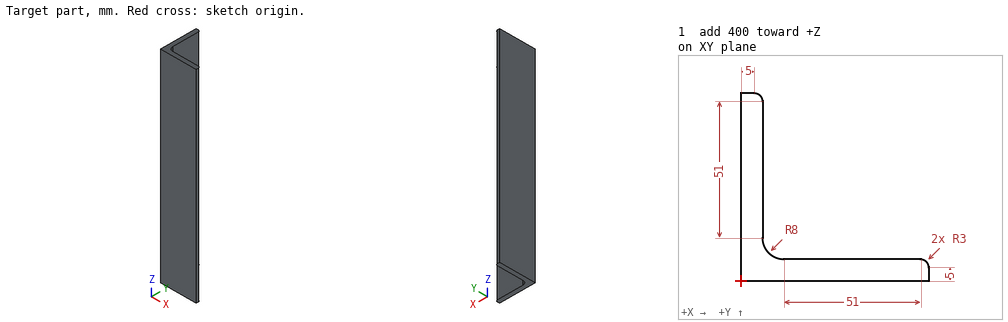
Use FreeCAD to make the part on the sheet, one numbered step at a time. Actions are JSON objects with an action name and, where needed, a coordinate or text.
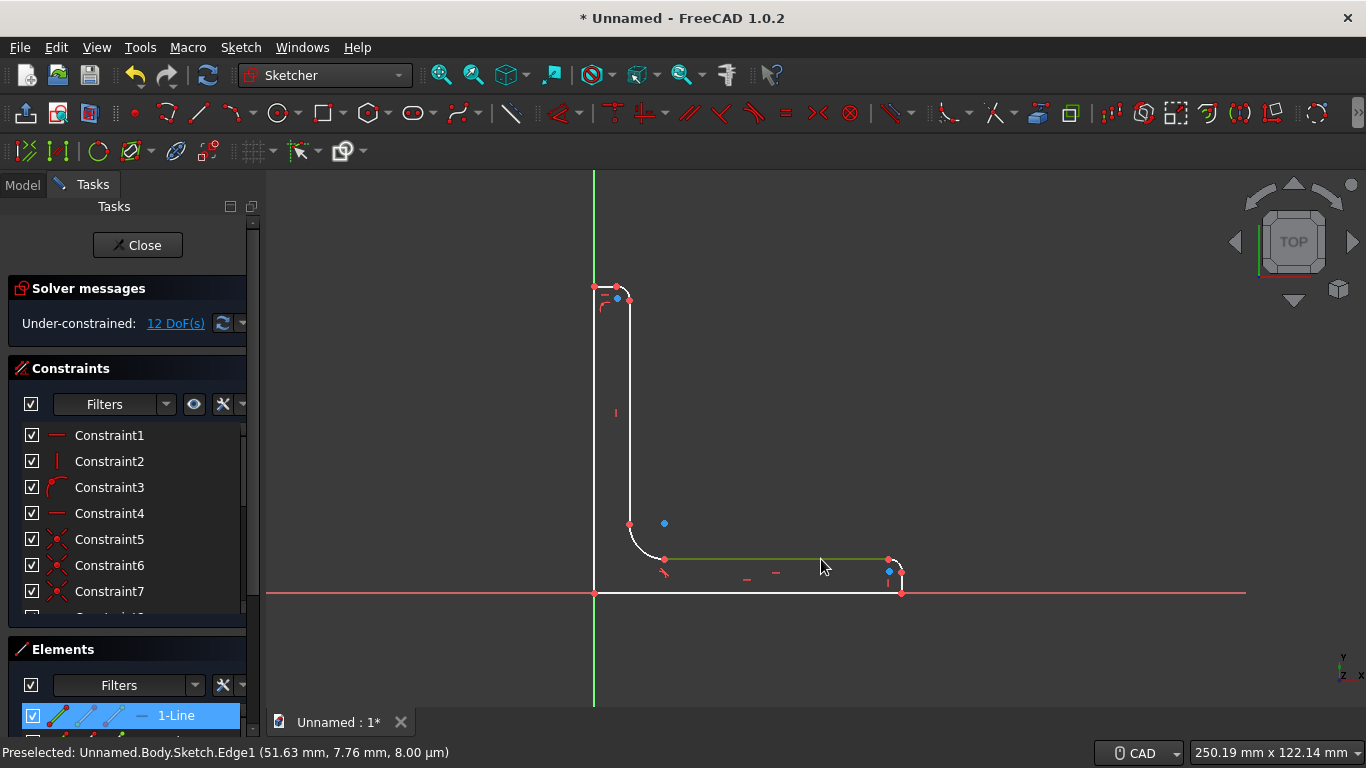
{"action": "scroll", "coordinate": [898, 563], "scroll_direction": "up", "scroll_amount": 2}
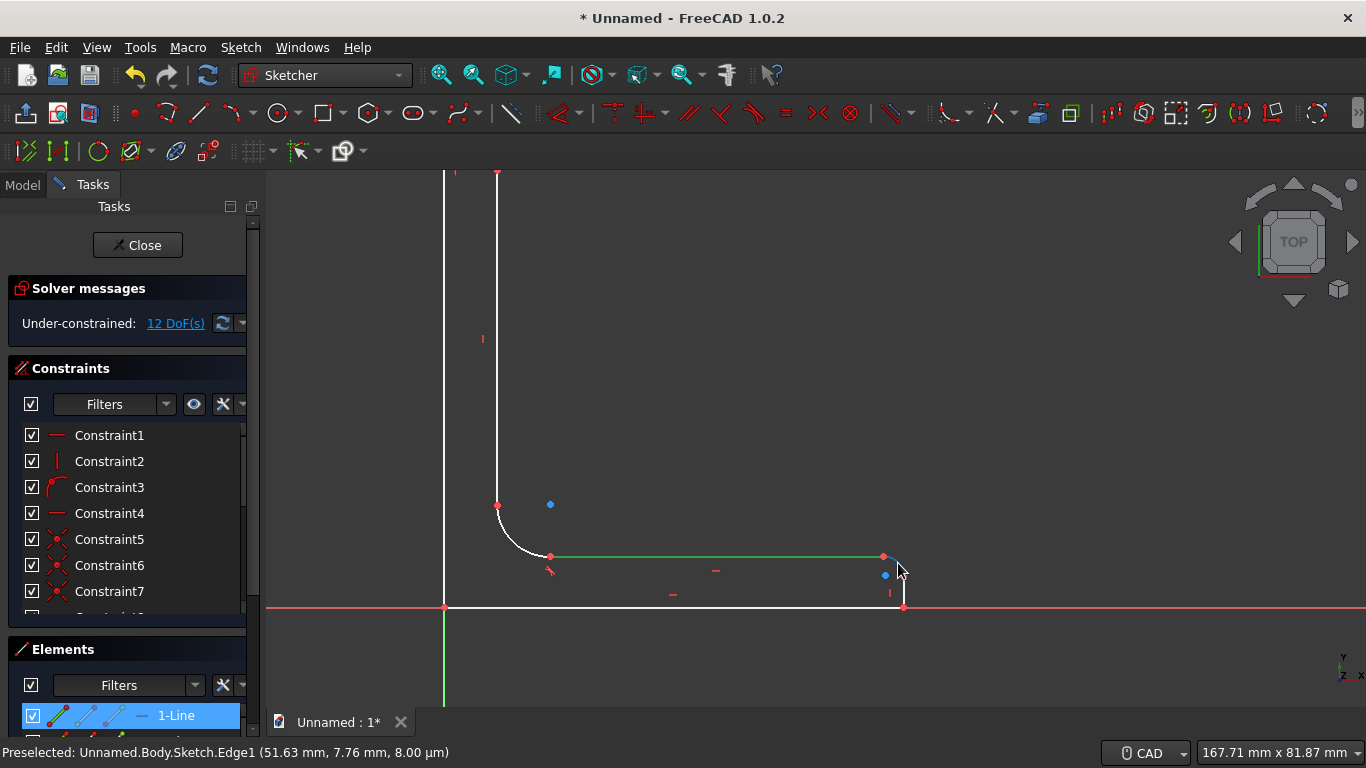
{"action": "left_click", "coordinate": [898, 562]}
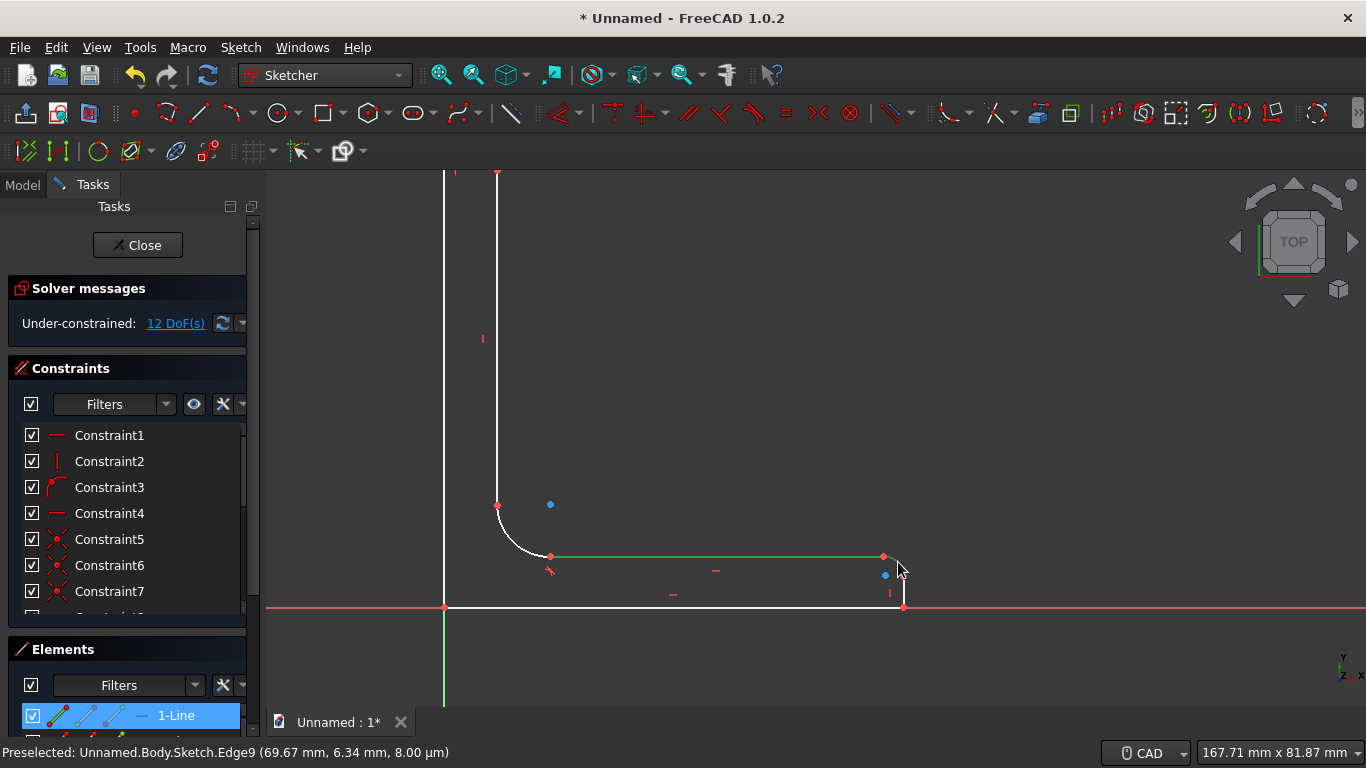
{"action": "left_click", "coordinate": [754, 114]}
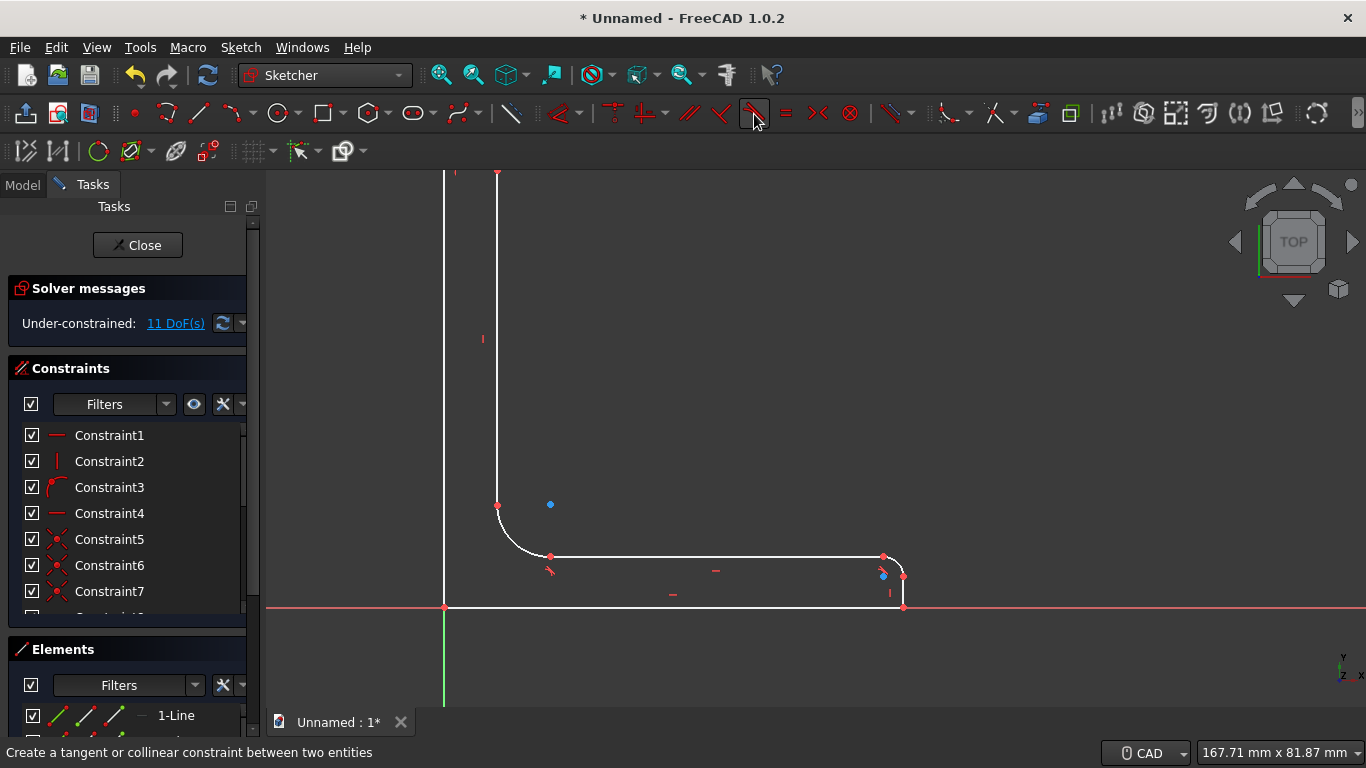
{"action": "left_click", "coordinate": [497, 405]}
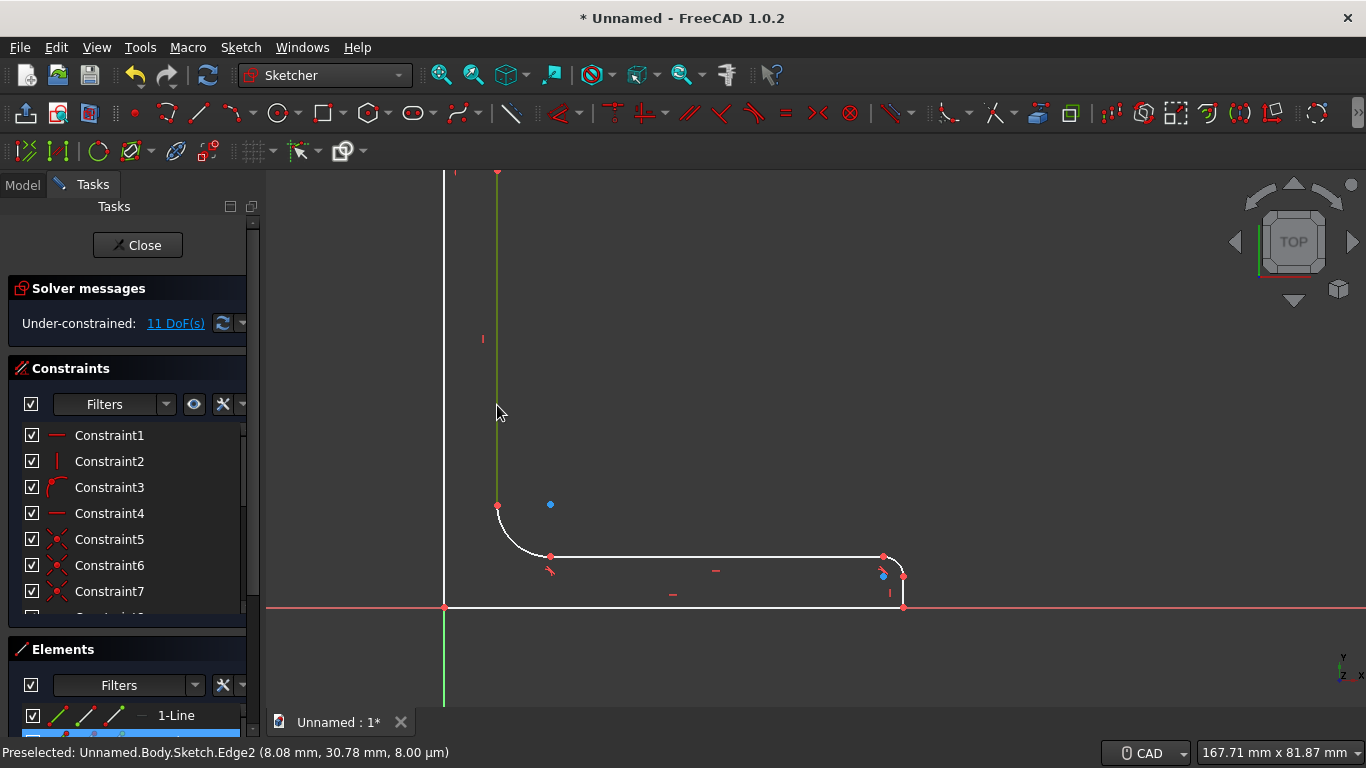
{"action": "left_click", "coordinate": [503, 529]}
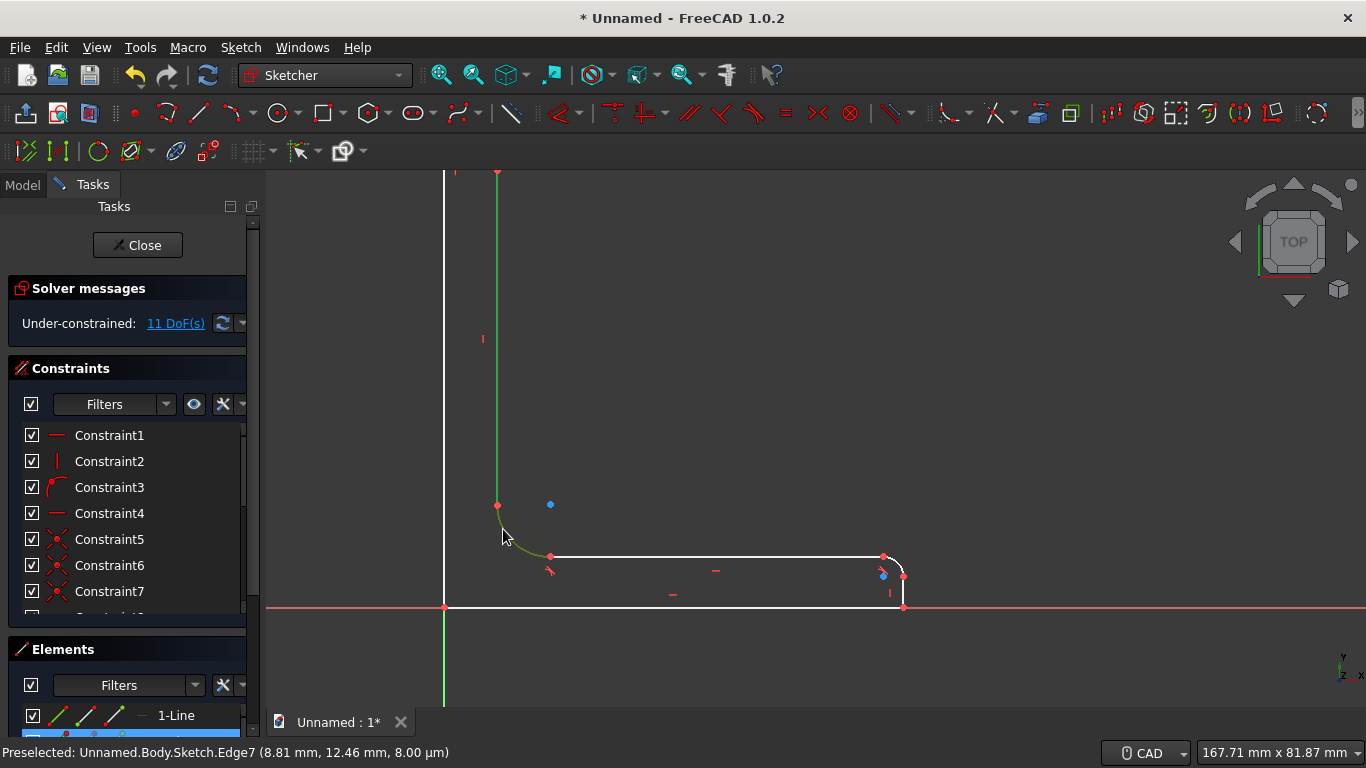
{"action": "left_click", "coordinate": [754, 114]}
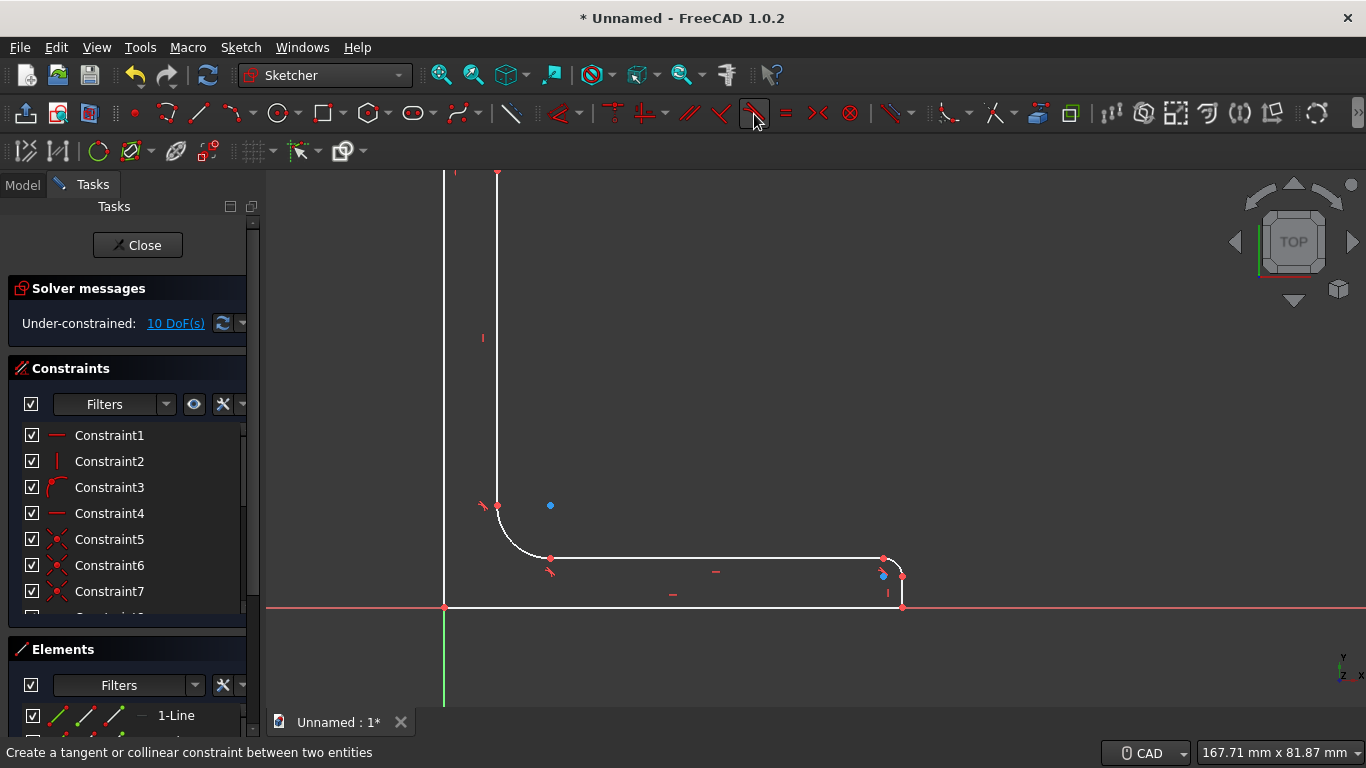
{"action": "left_click", "coordinate": [497, 405]}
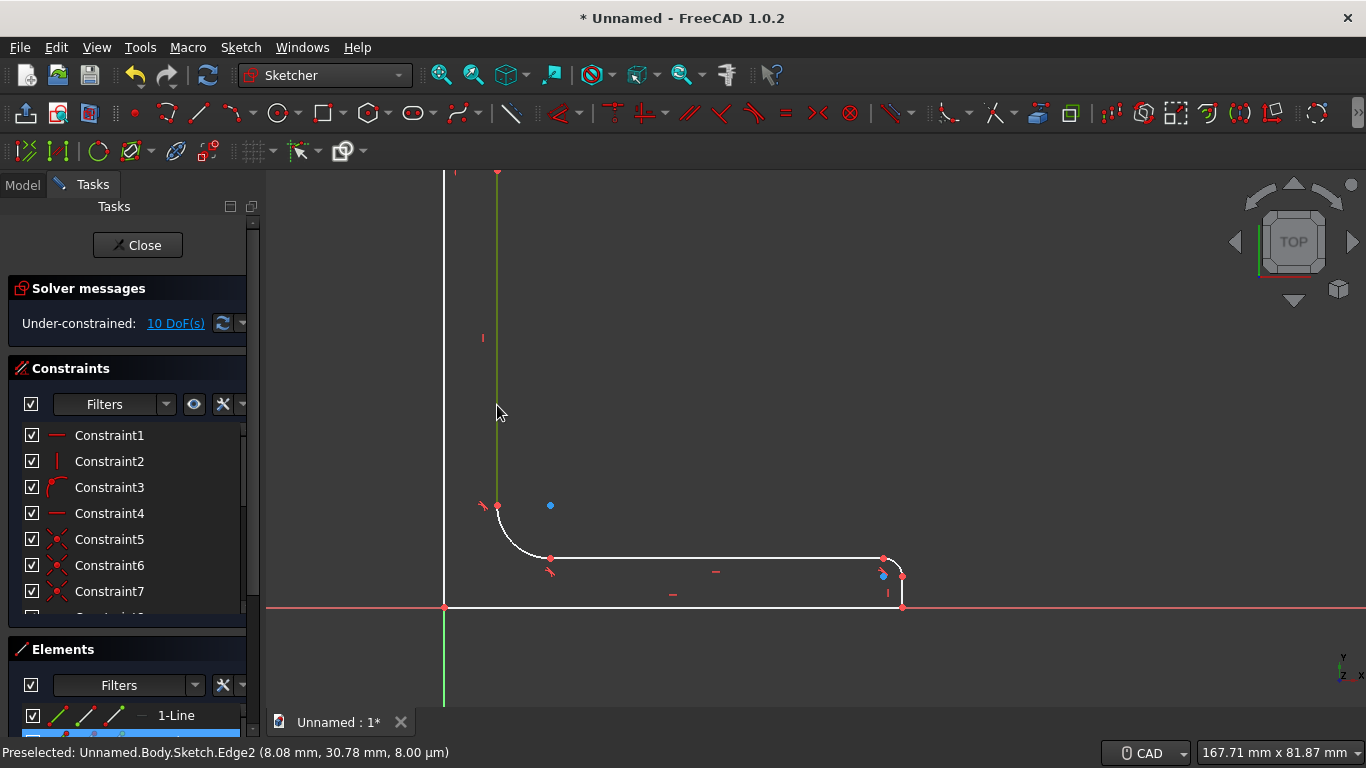
{"action": "scroll", "coordinate": [897, 561], "scroll_direction": "down", "scroll_amount": 2}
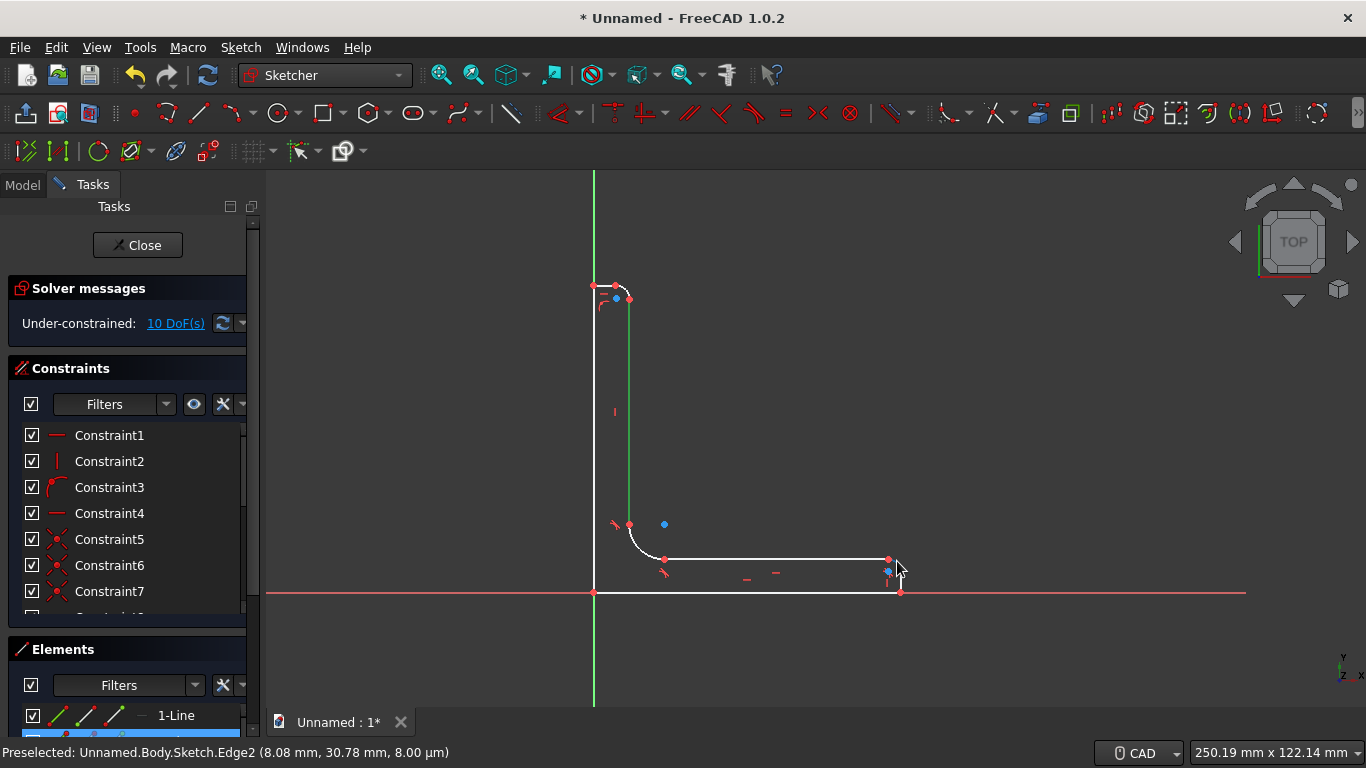
{"action": "scroll", "coordinate": [628, 293], "scroll_direction": "up", "scroll_amount": 4}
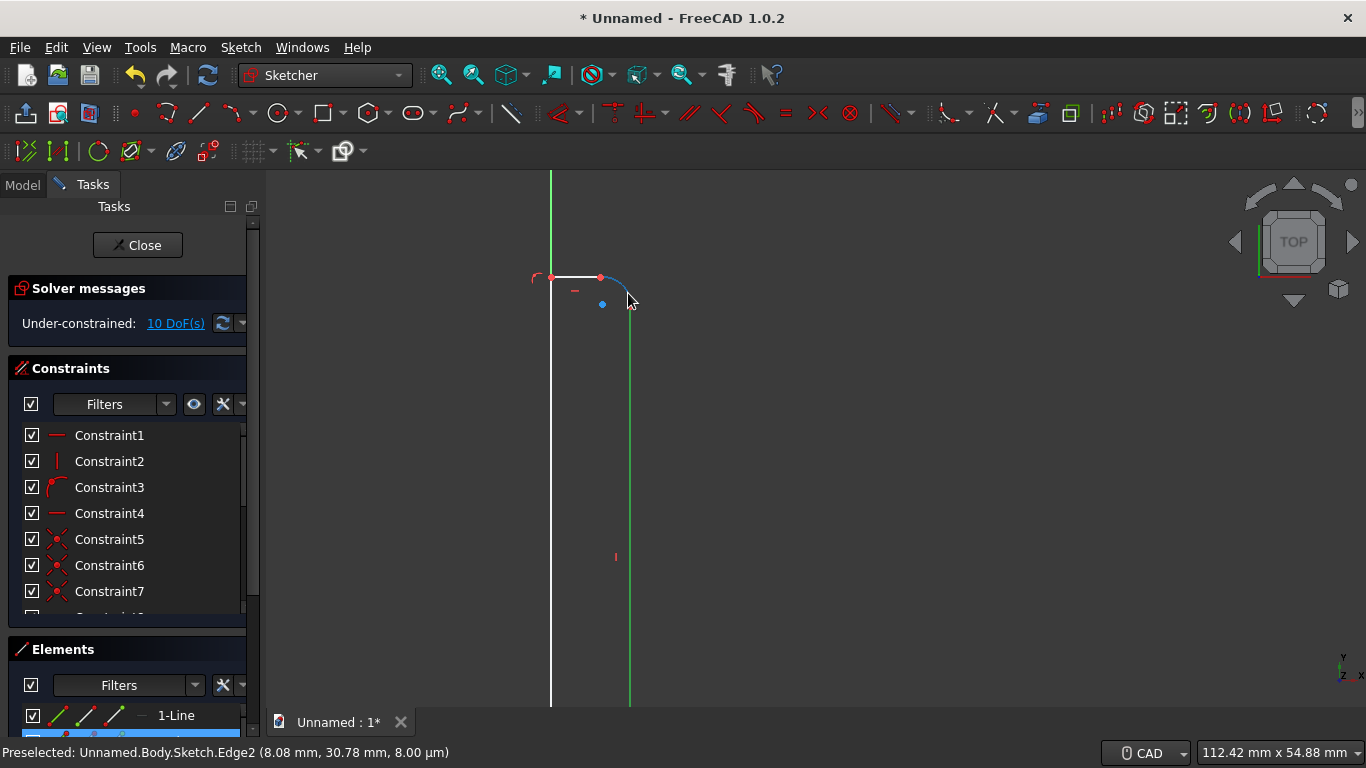
{"action": "left_click", "coordinate": [628, 293]}